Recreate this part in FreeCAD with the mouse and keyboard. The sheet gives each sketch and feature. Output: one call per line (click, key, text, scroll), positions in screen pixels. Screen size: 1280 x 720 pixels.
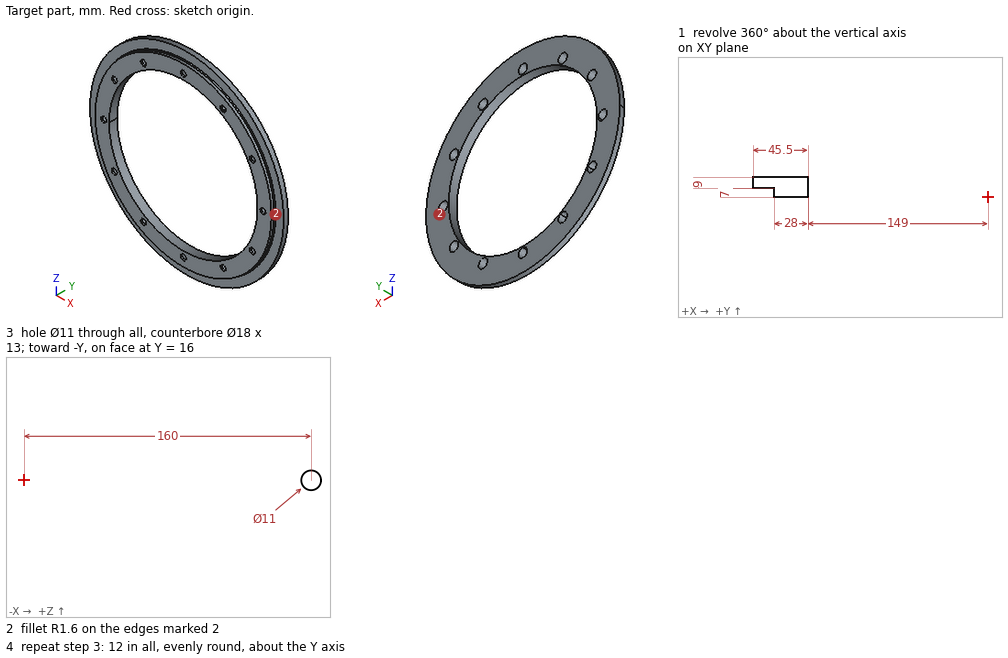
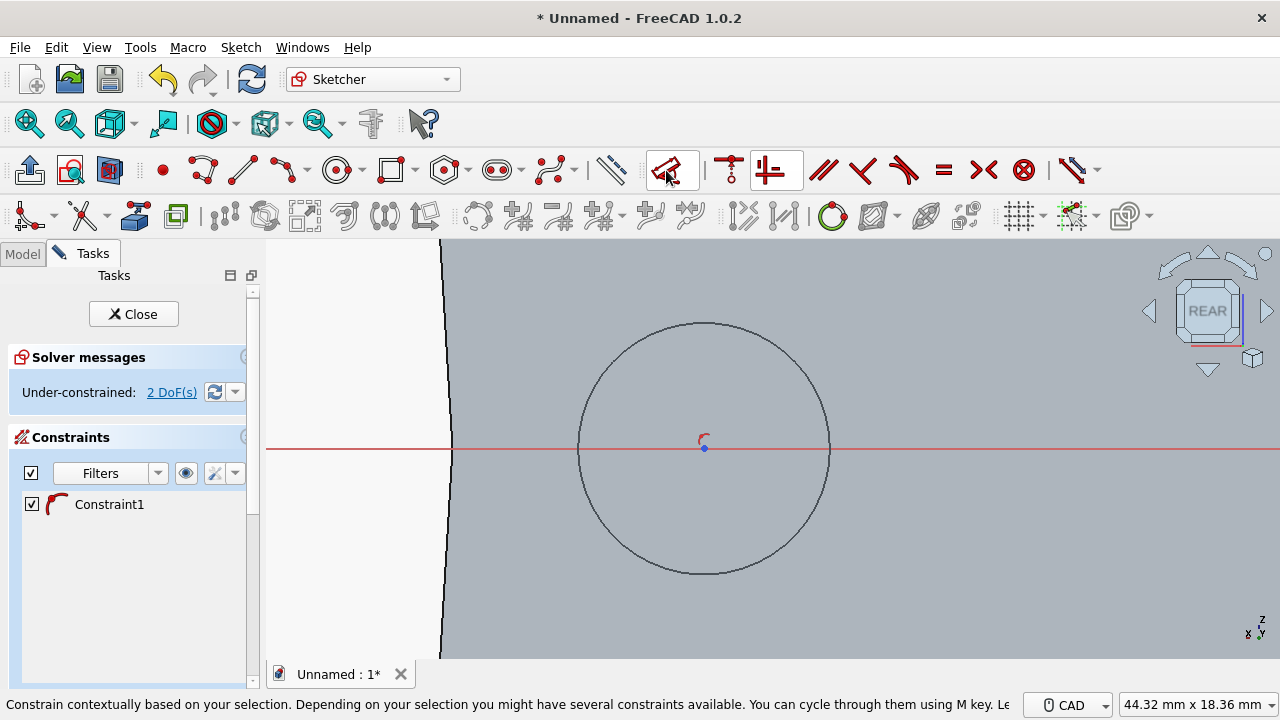
click(793, 360)
click(816, 337)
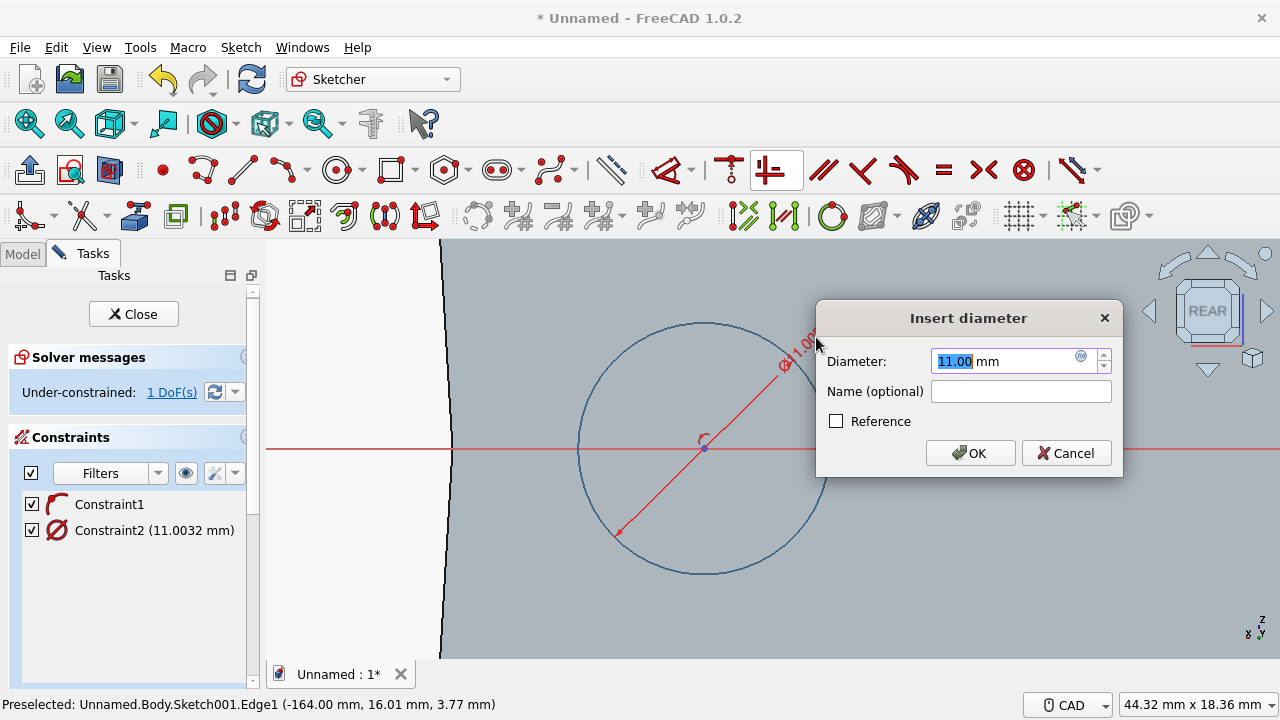
text(11)
key(Return)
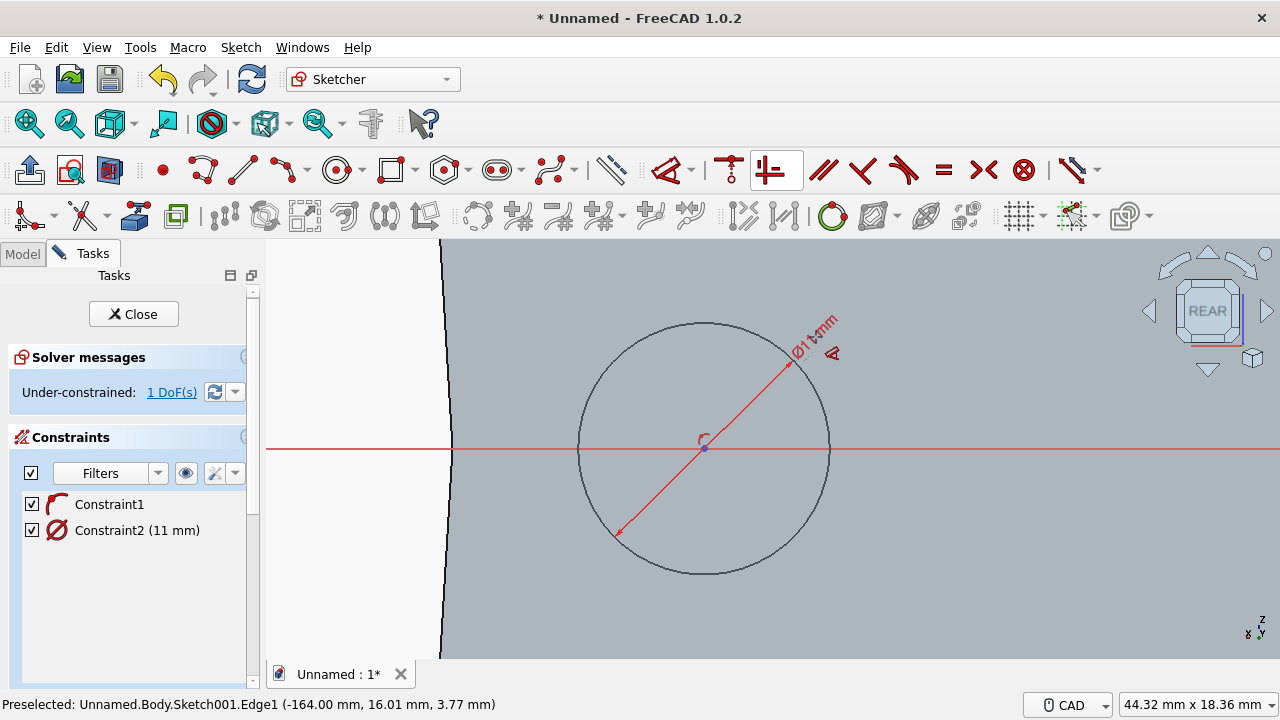
click(704, 449)
click(499, 483)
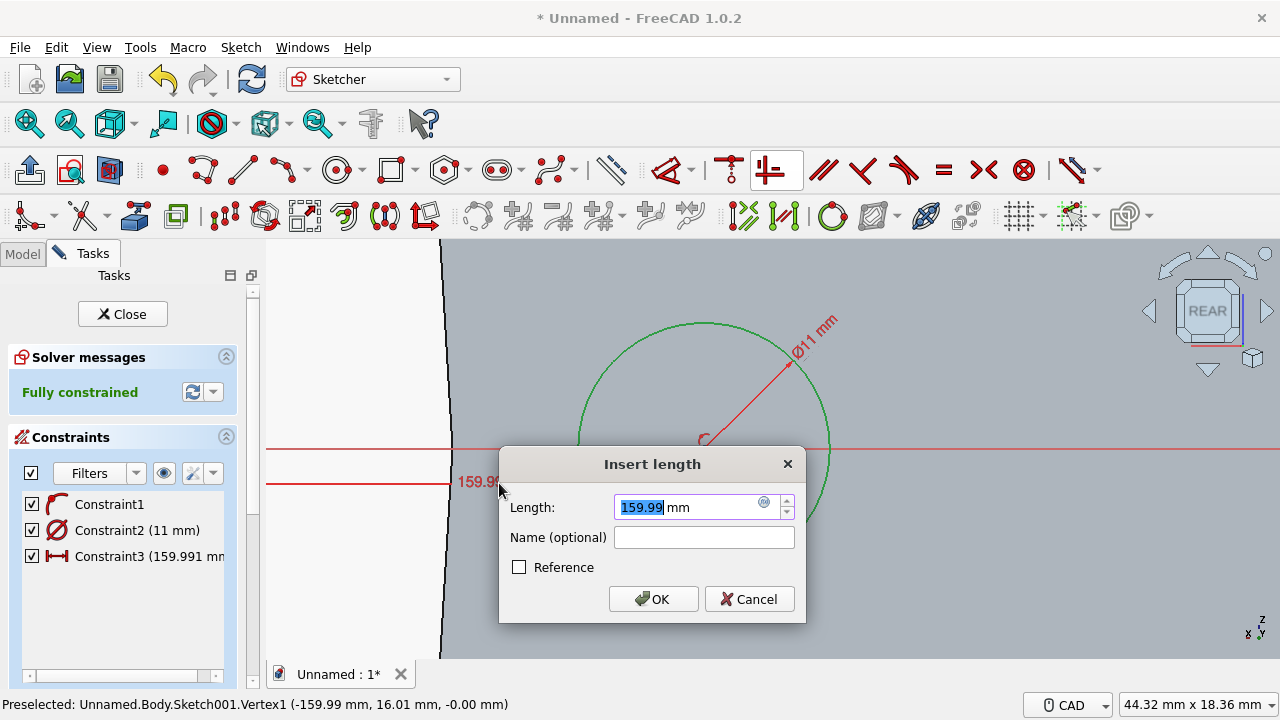
text(160)
key(Return)
key(Escape)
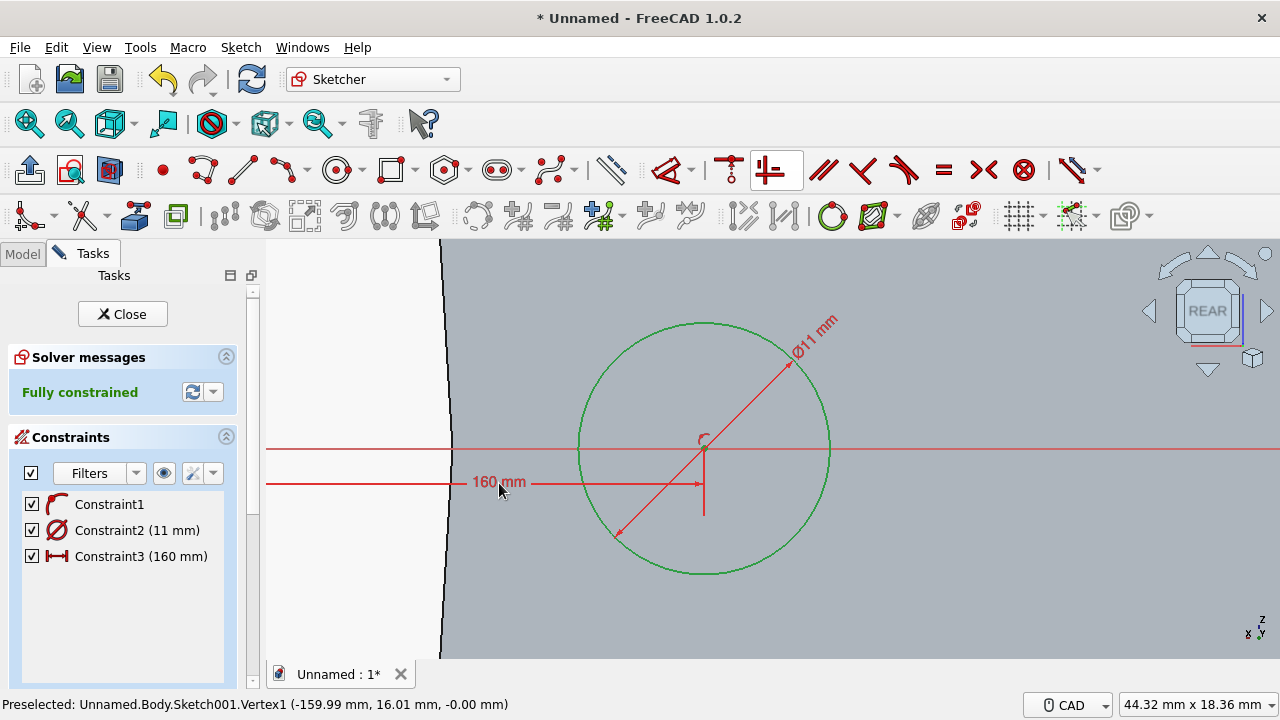
click(123, 314)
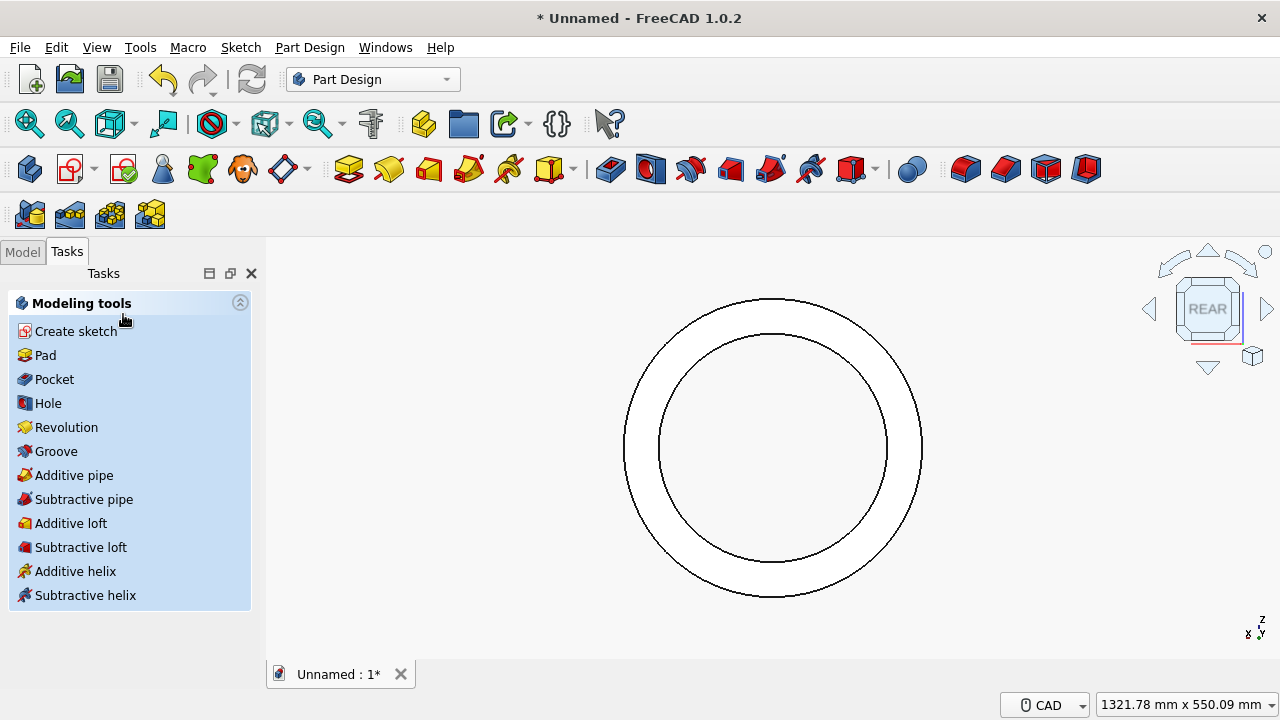
click(652, 170)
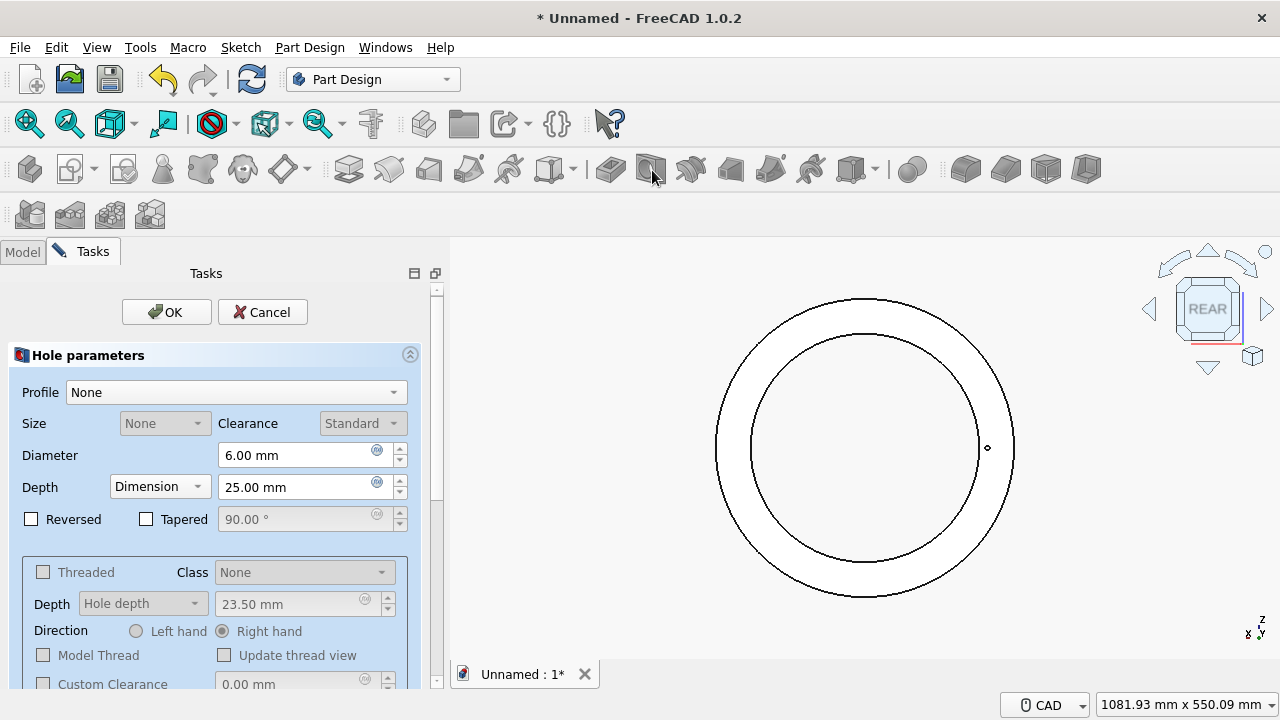
triple_click(305, 455)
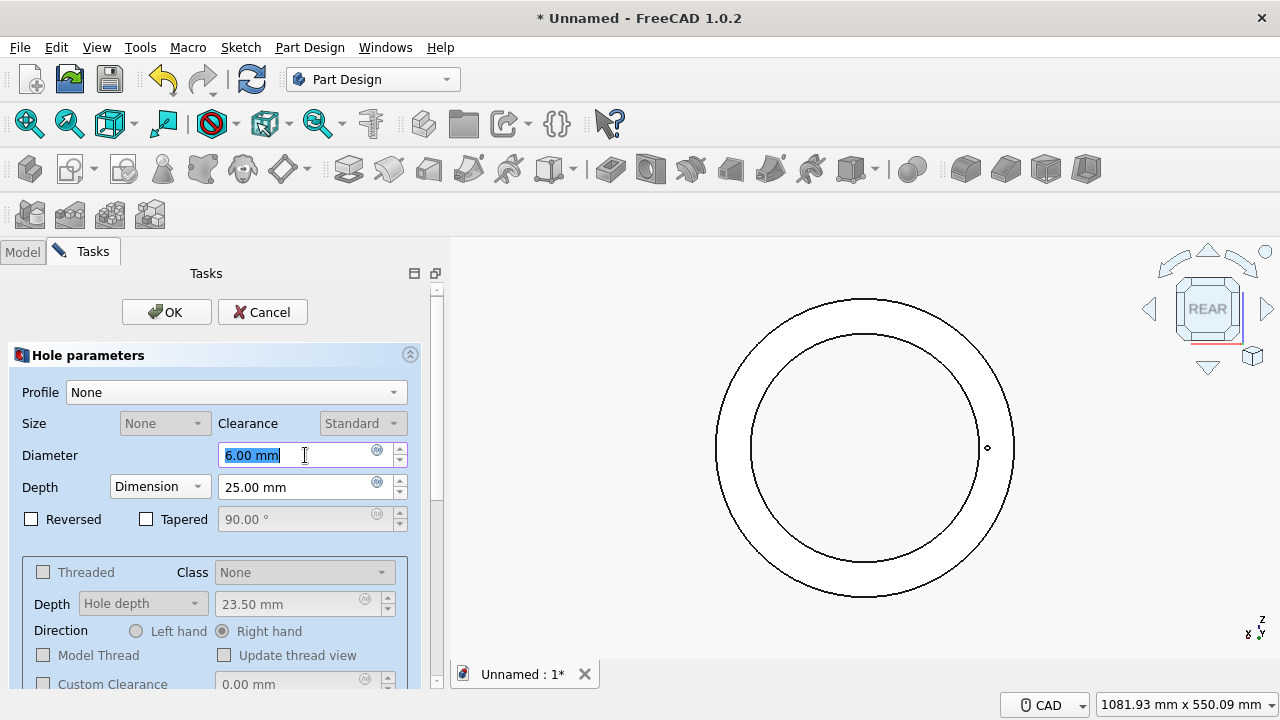
text(11)
key(Tab)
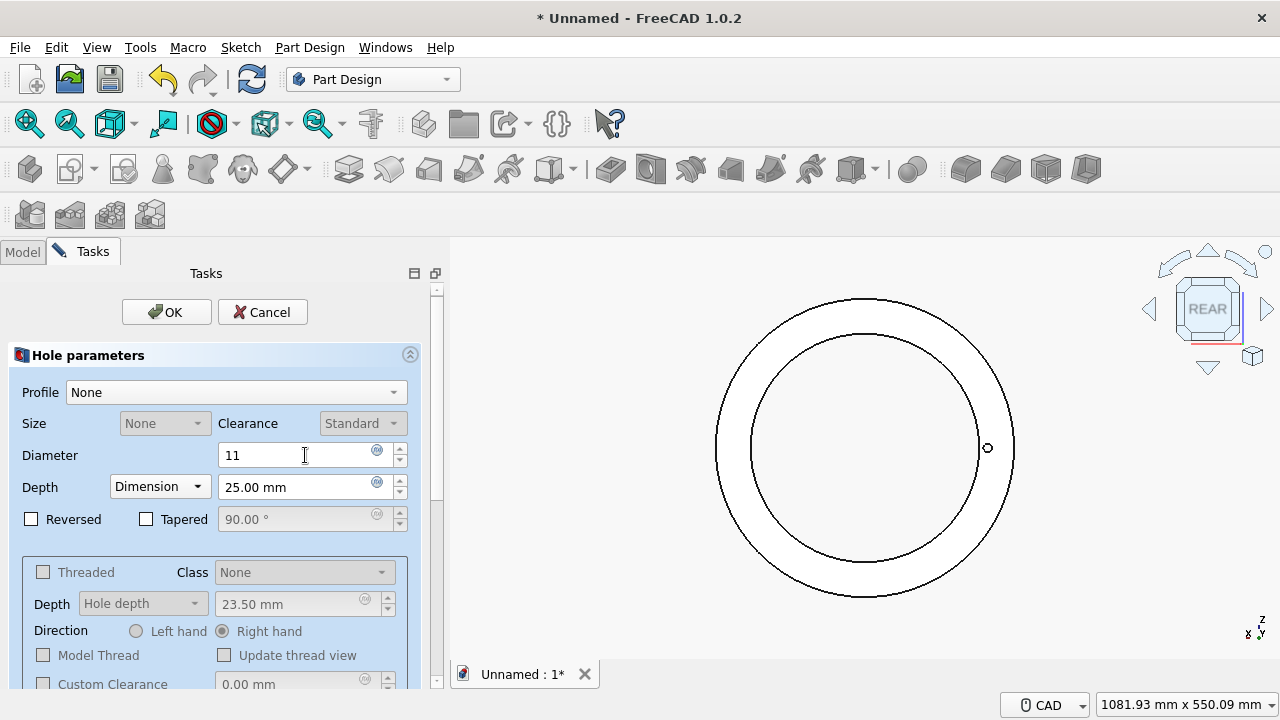
click(161, 486)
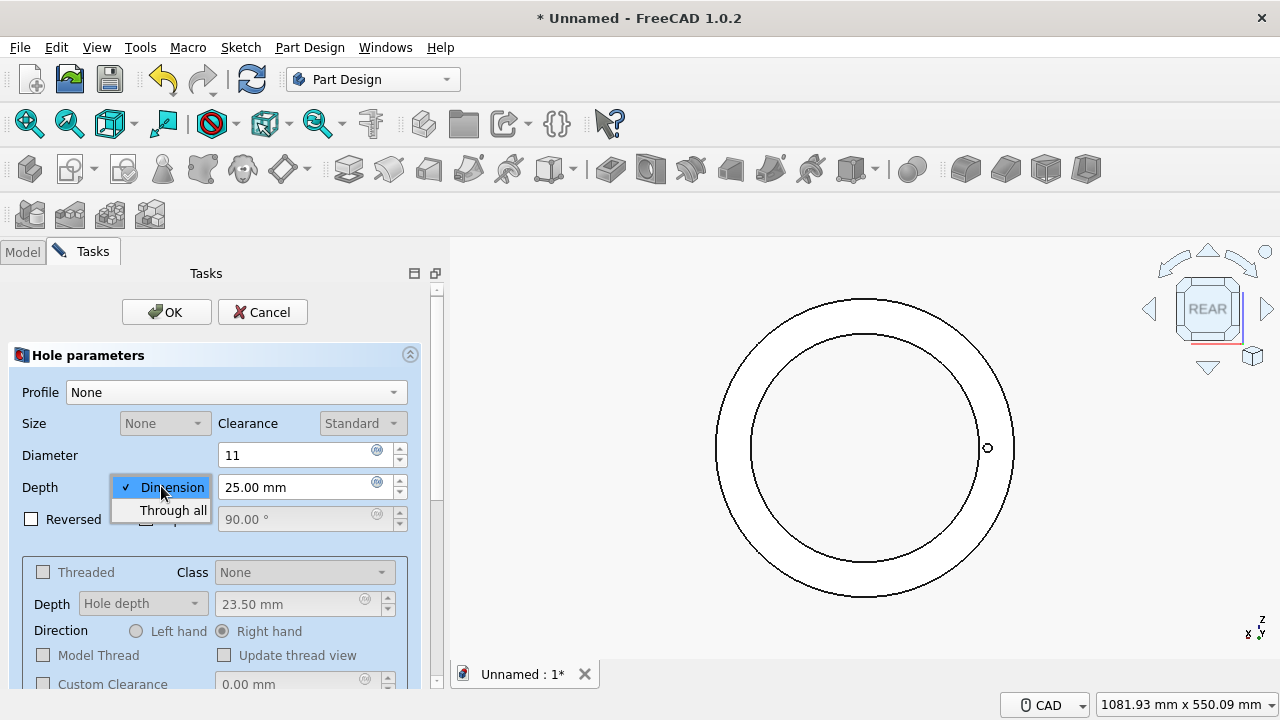
click(160, 510)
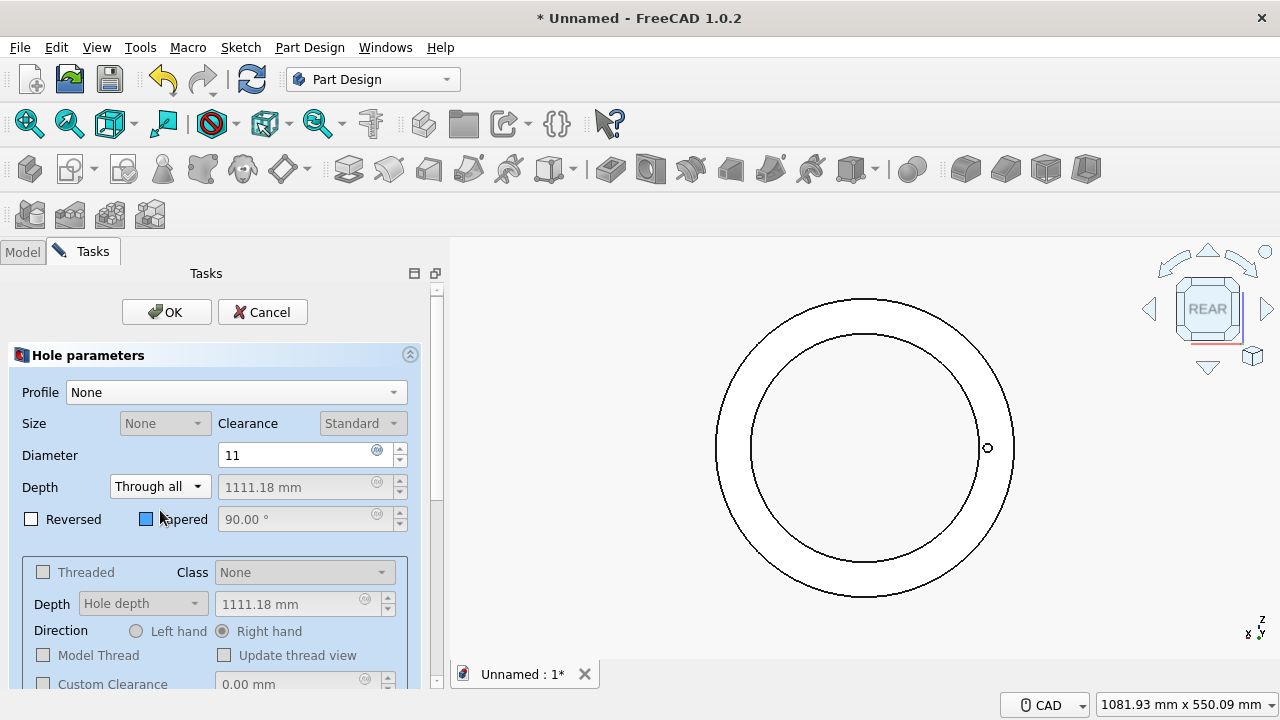
scroll(437, 486, down, 3)